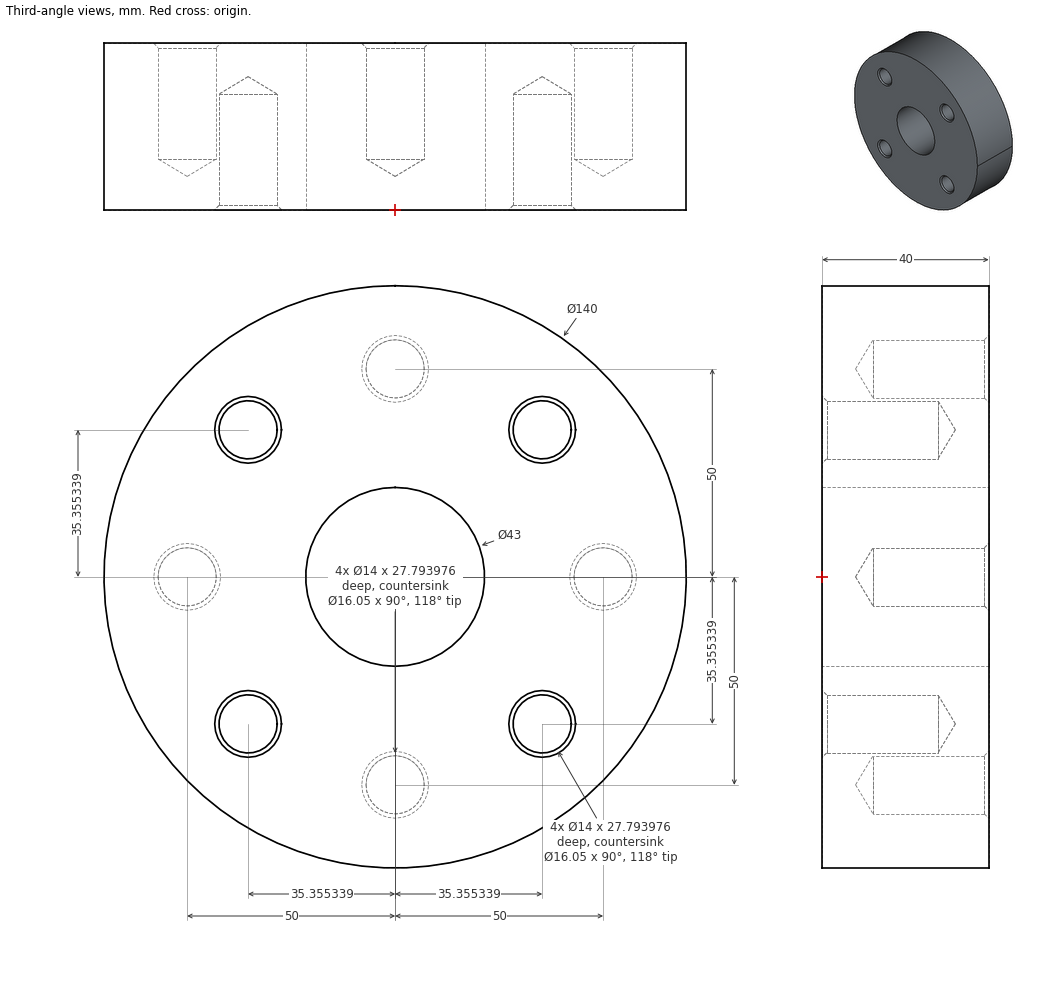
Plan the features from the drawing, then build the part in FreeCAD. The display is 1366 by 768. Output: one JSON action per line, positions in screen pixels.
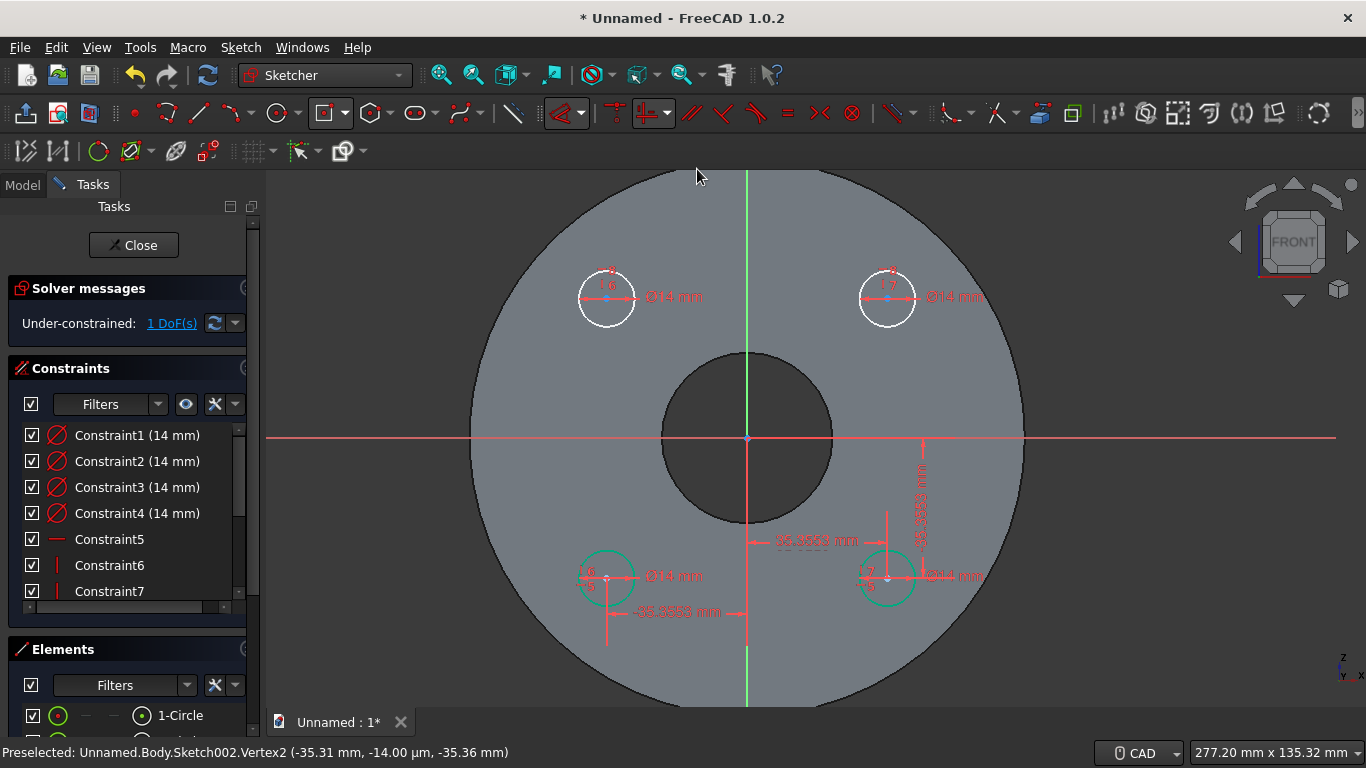
{"action": "left_click", "coordinate": [607, 299]}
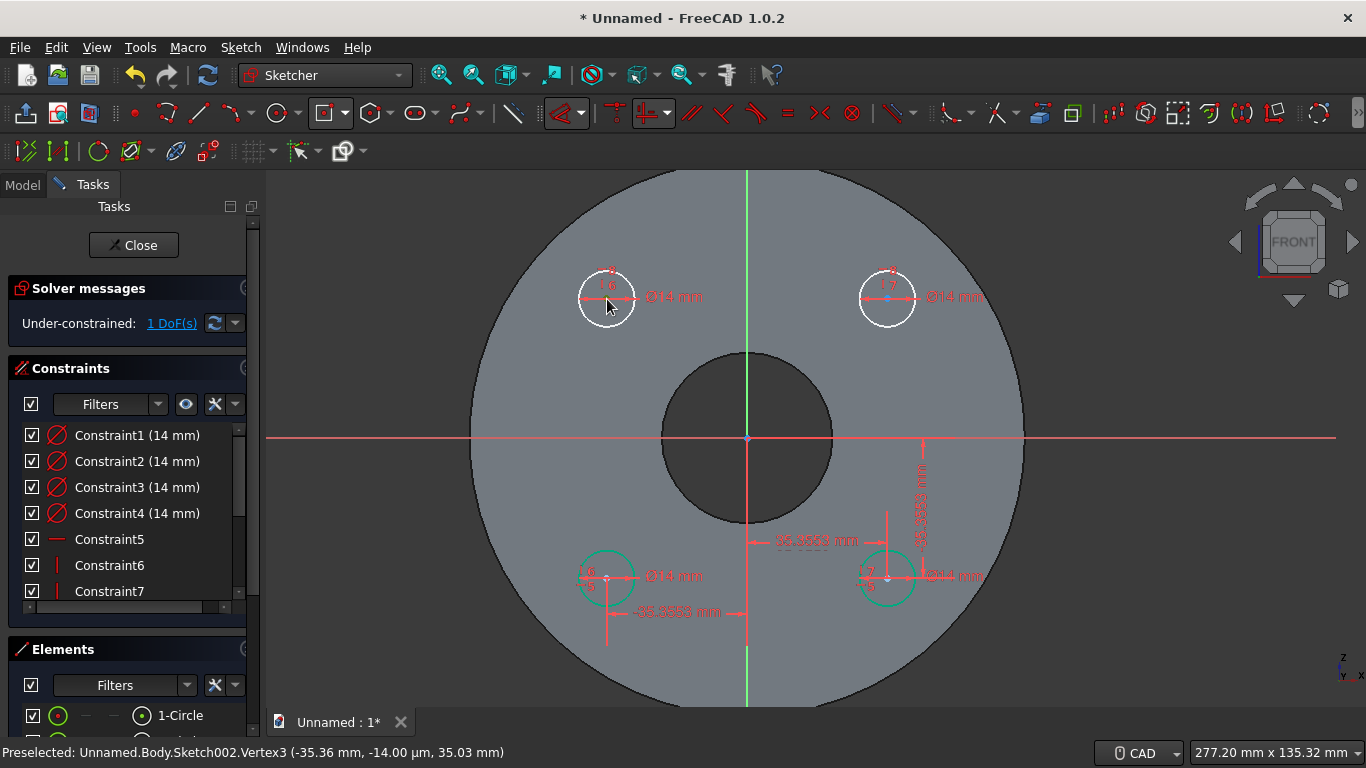
{"action": "key", "text": "i"}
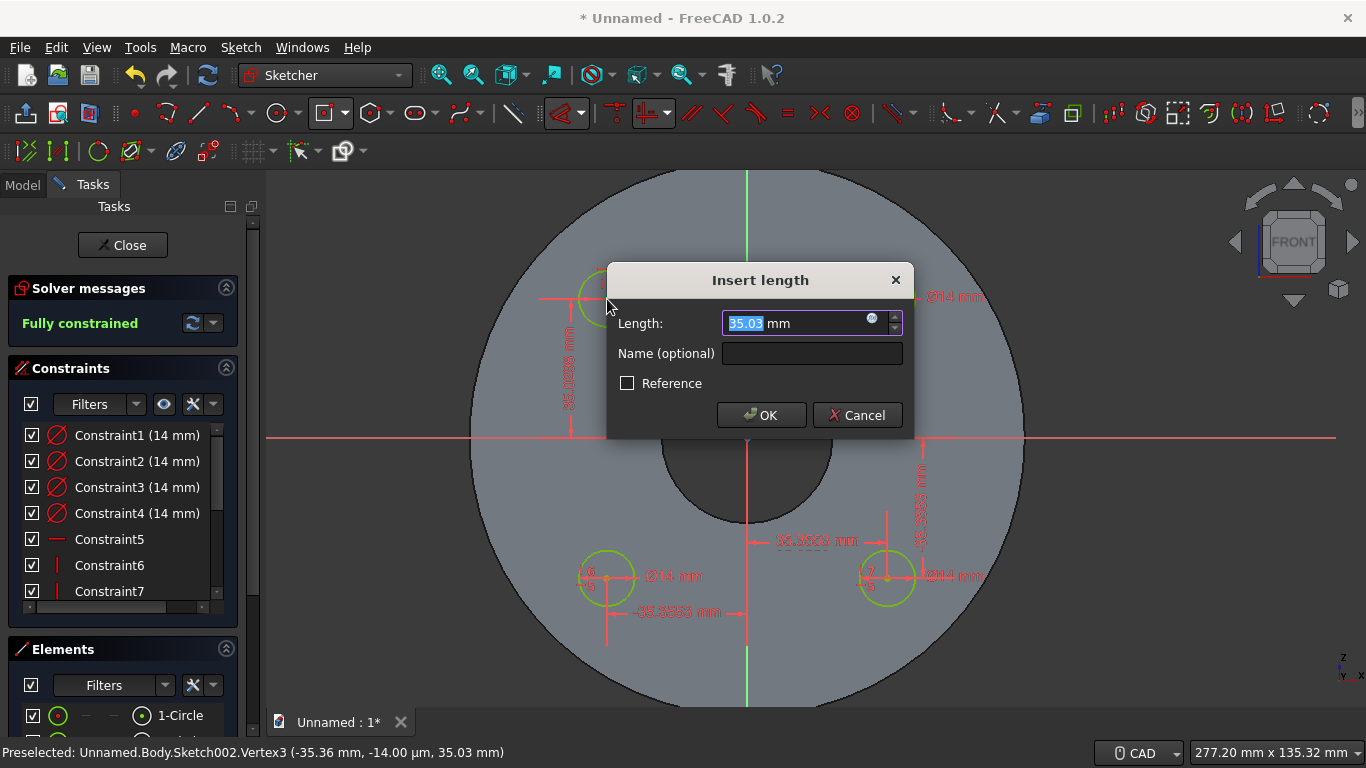
{"action": "type", "text": "35.355339"}
{"action": "key", "text": "Return"}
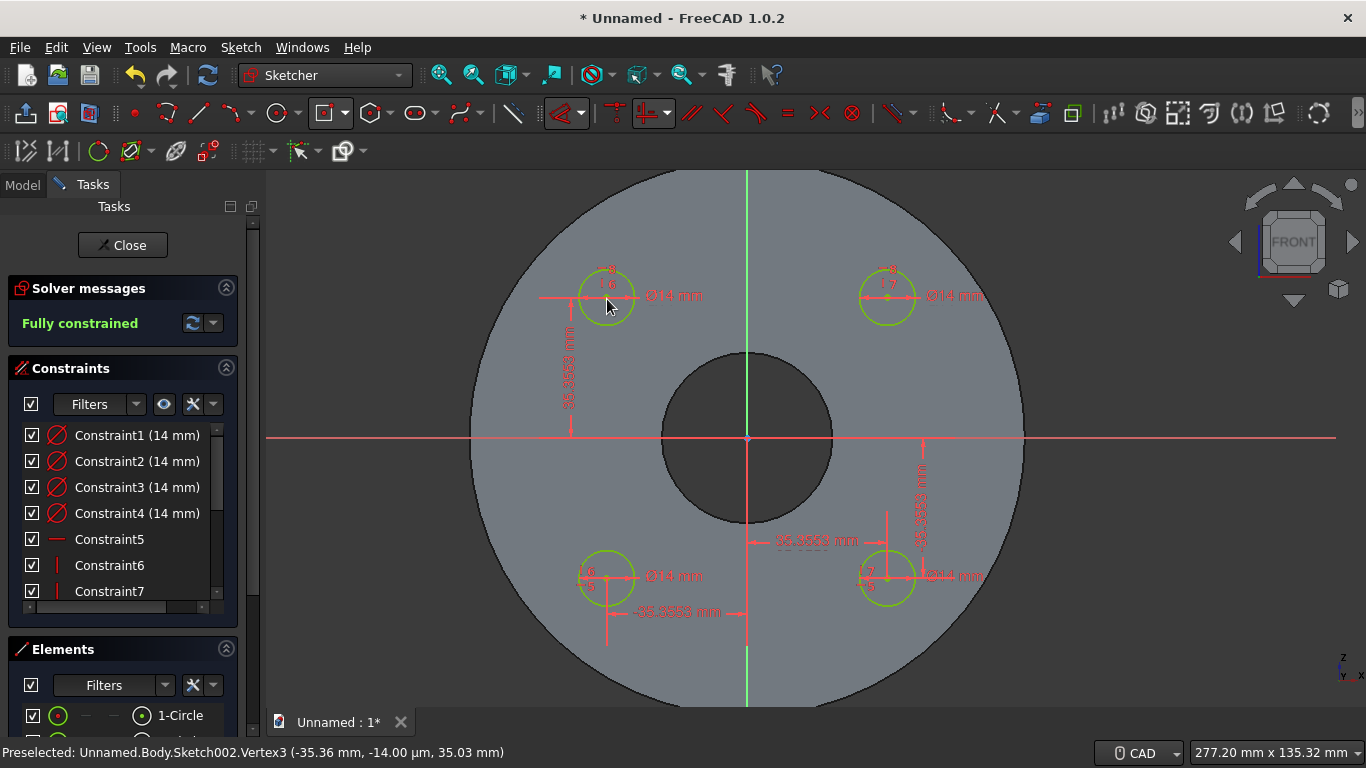
{"action": "left_click", "coordinate": [123, 245]}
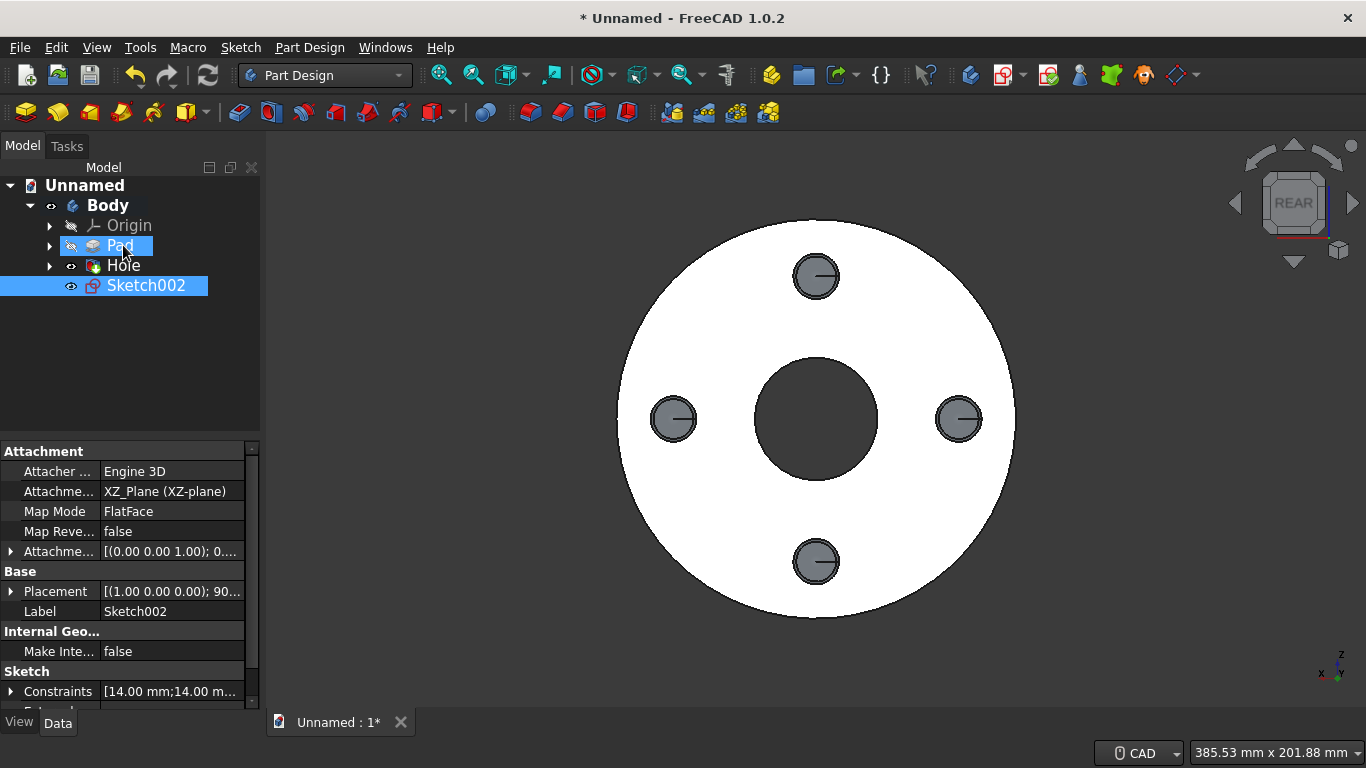
{"action": "left_click", "coordinate": [272, 112]}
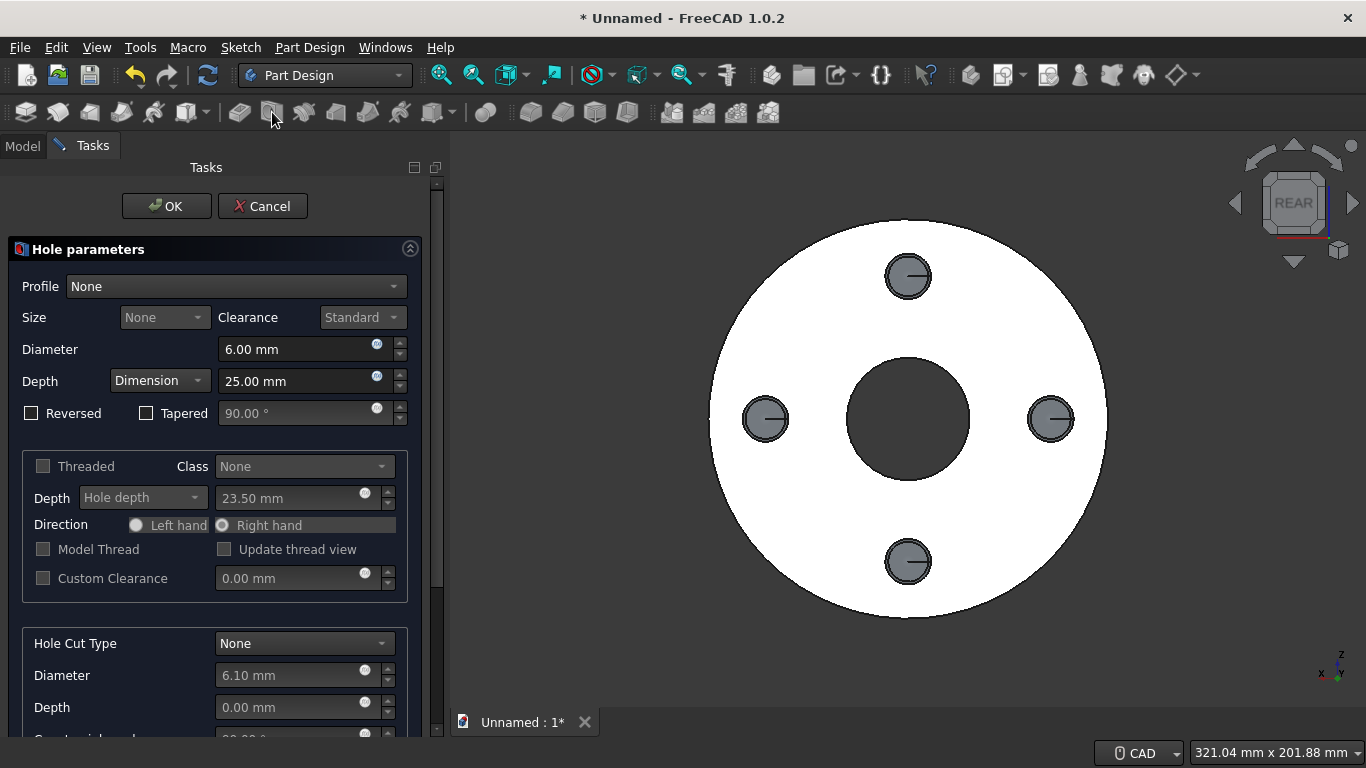
{"action": "triple_click", "coordinate": [305, 349]}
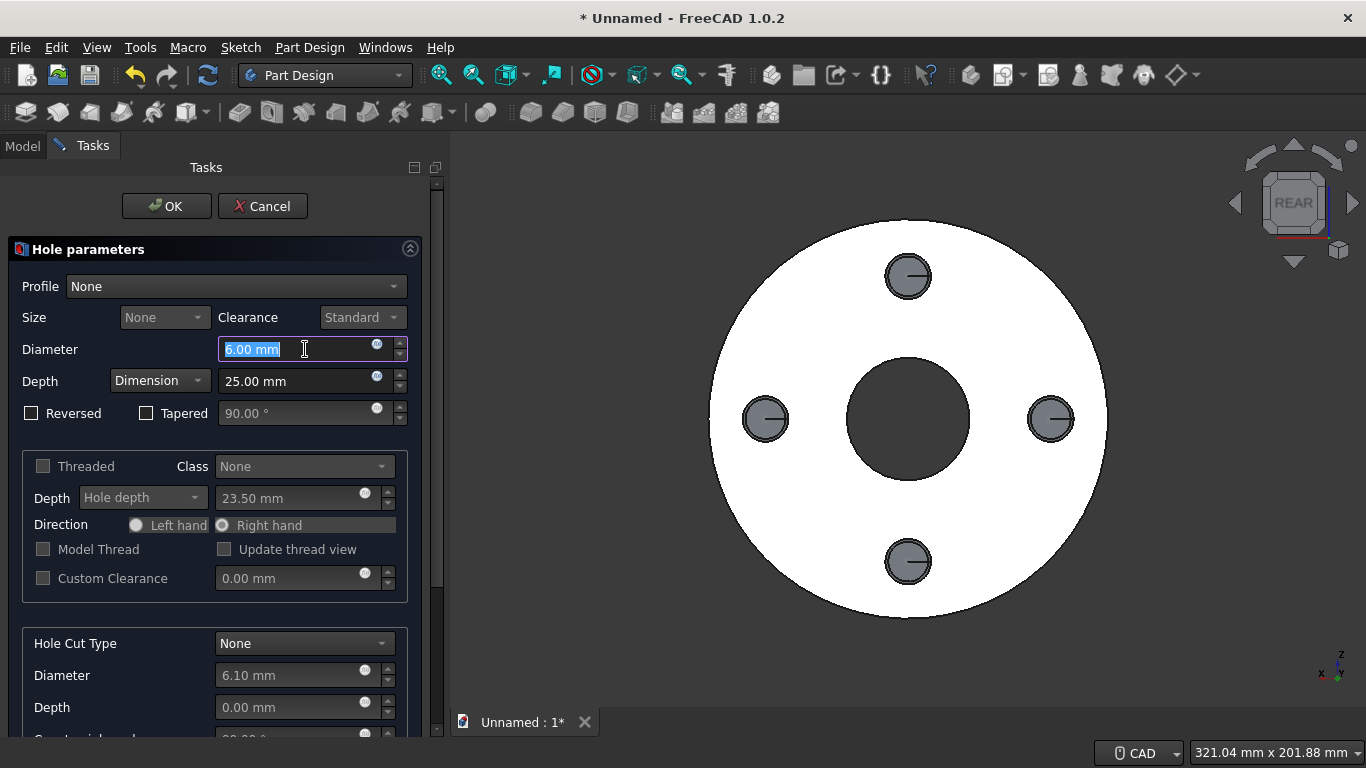
{"action": "type", "text": "14"}
{"action": "key", "text": "Tab"}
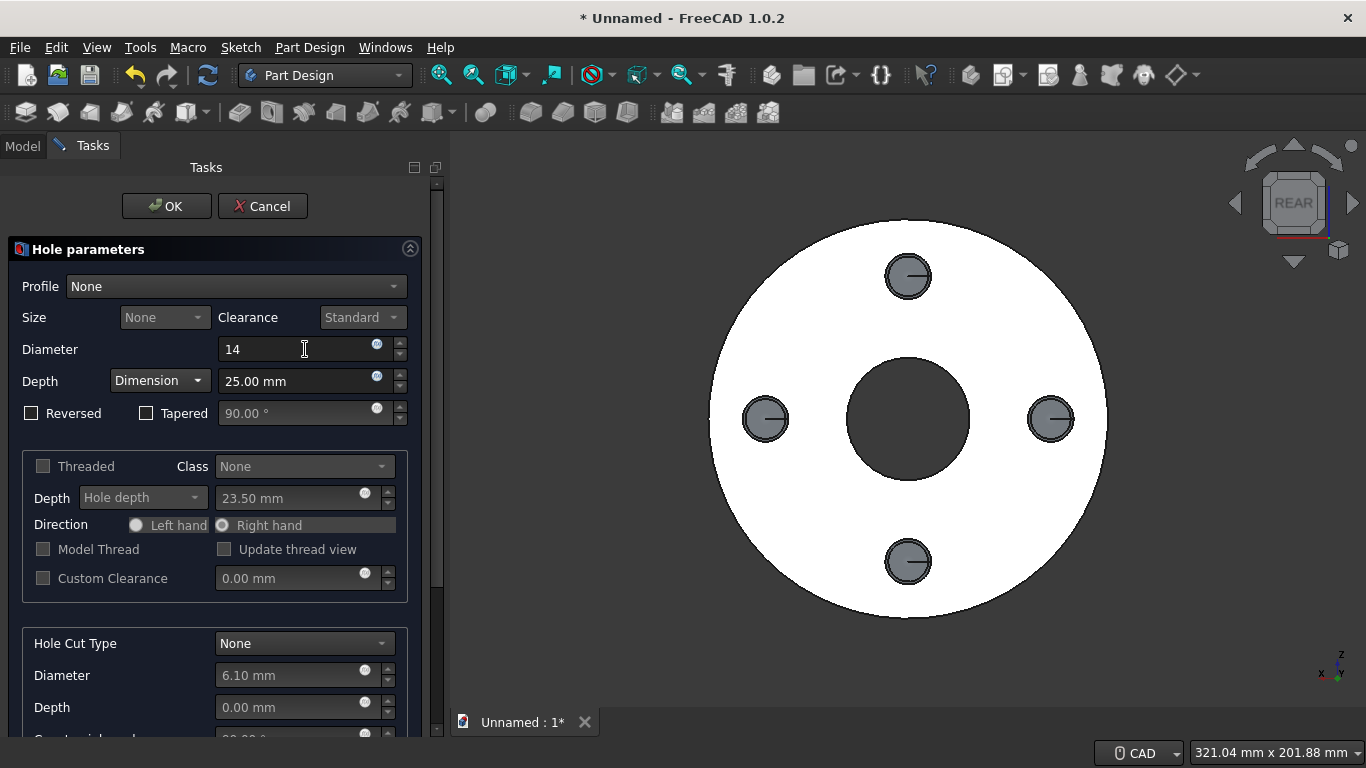
{"action": "triple_click", "coordinate": [305, 381]}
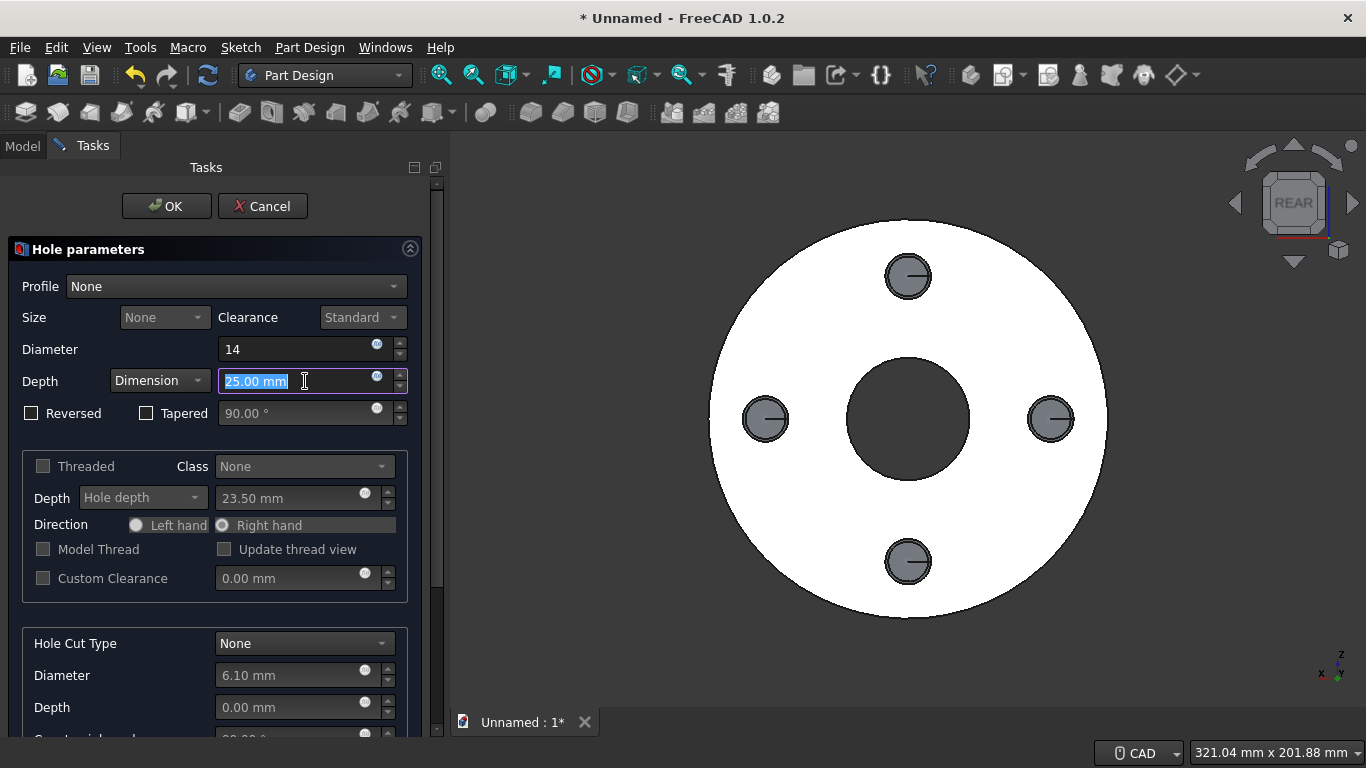
{"action": "type", "text": "27.793976"}
{"action": "key", "text": "Tab"}